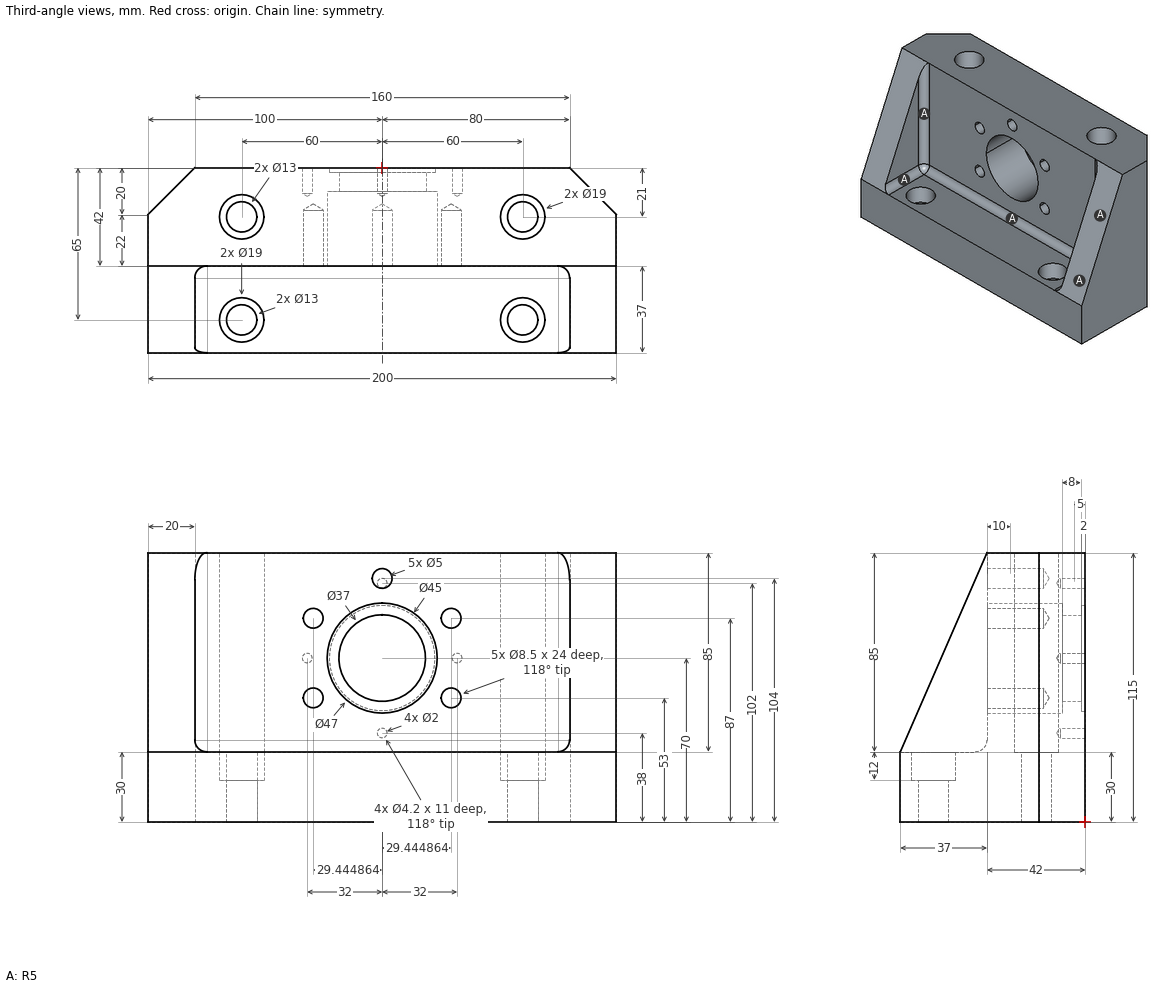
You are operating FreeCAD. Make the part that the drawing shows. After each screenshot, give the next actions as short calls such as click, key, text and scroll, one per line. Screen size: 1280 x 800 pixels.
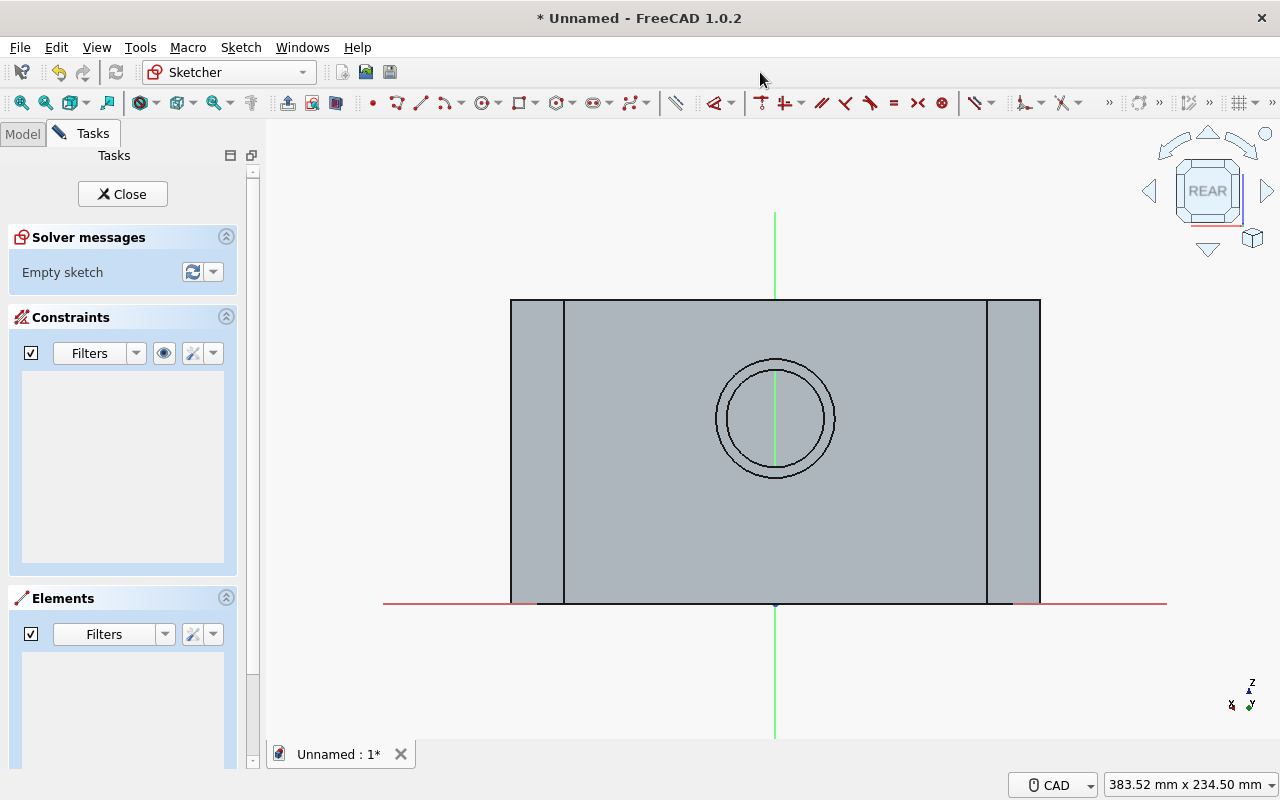
click(336, 104)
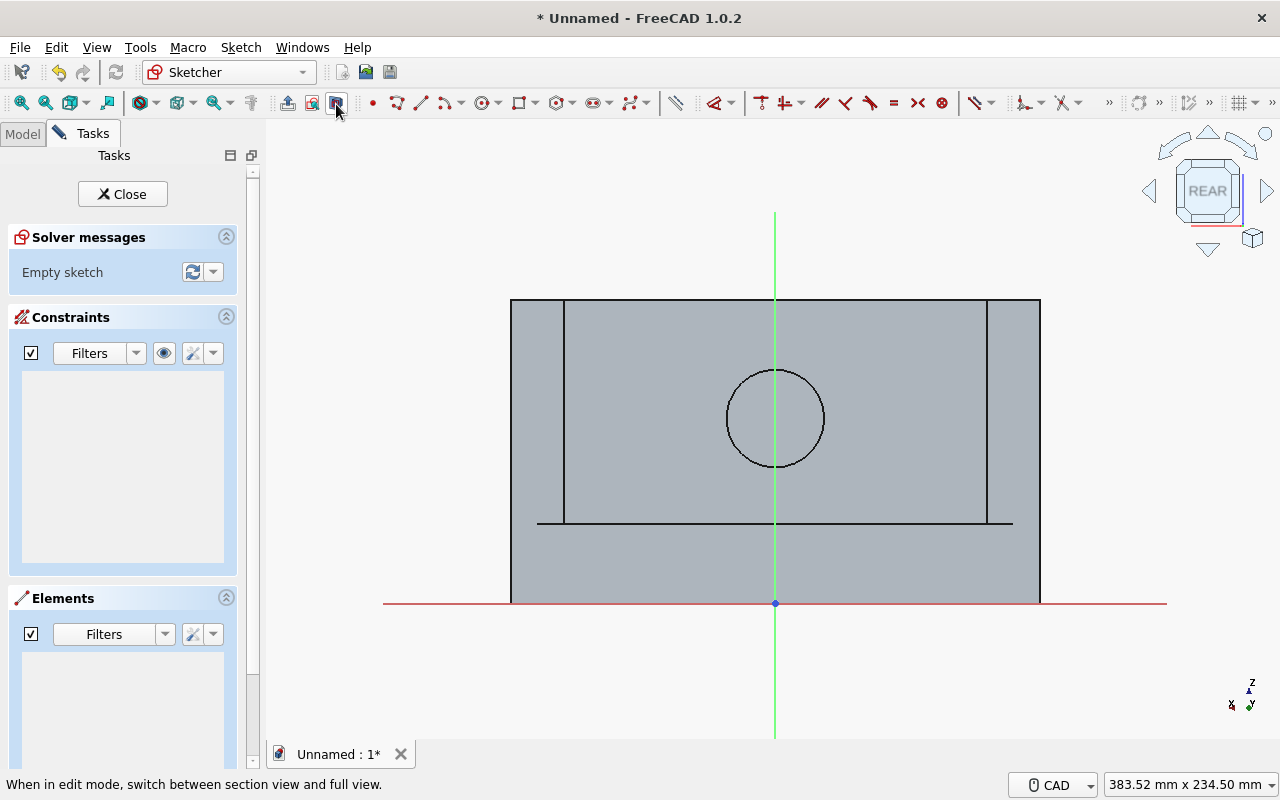
scroll(919, 584, up, 2)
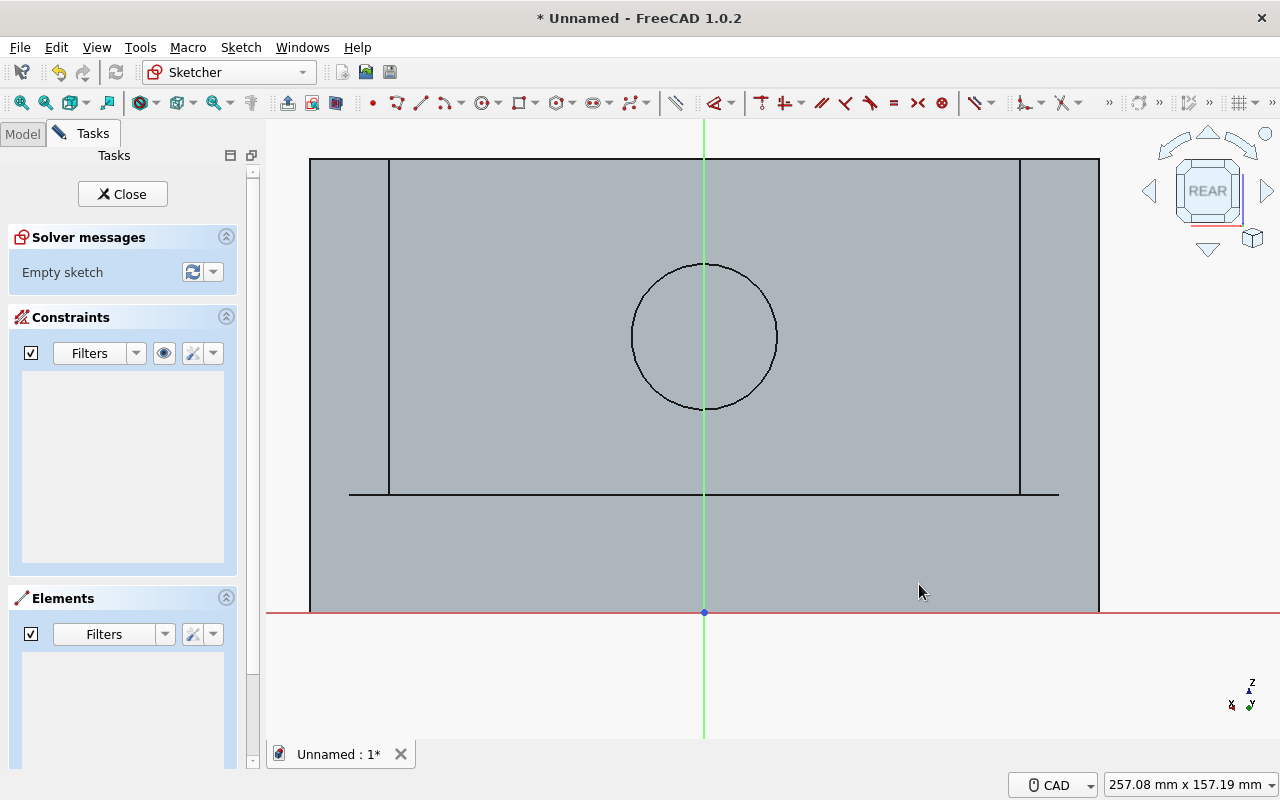
click(482, 104)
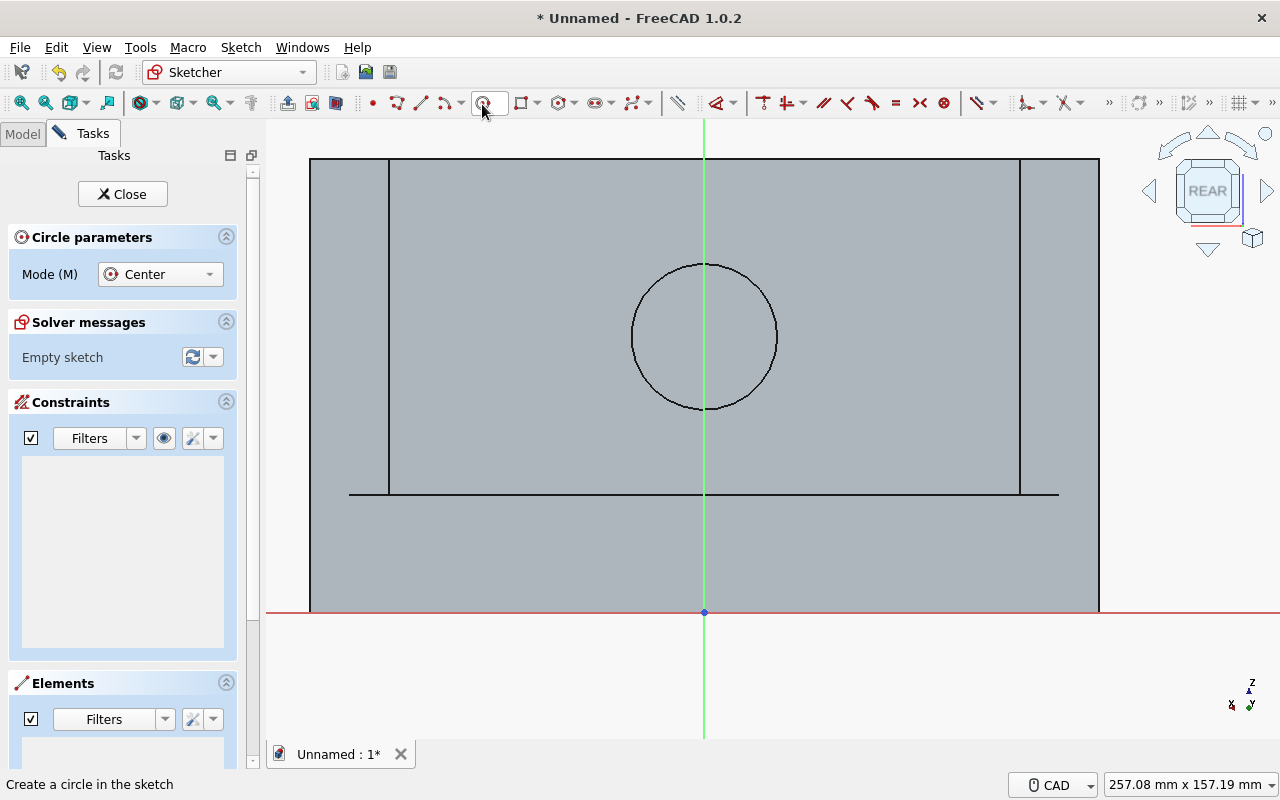
click(704, 337)
move(770, 271)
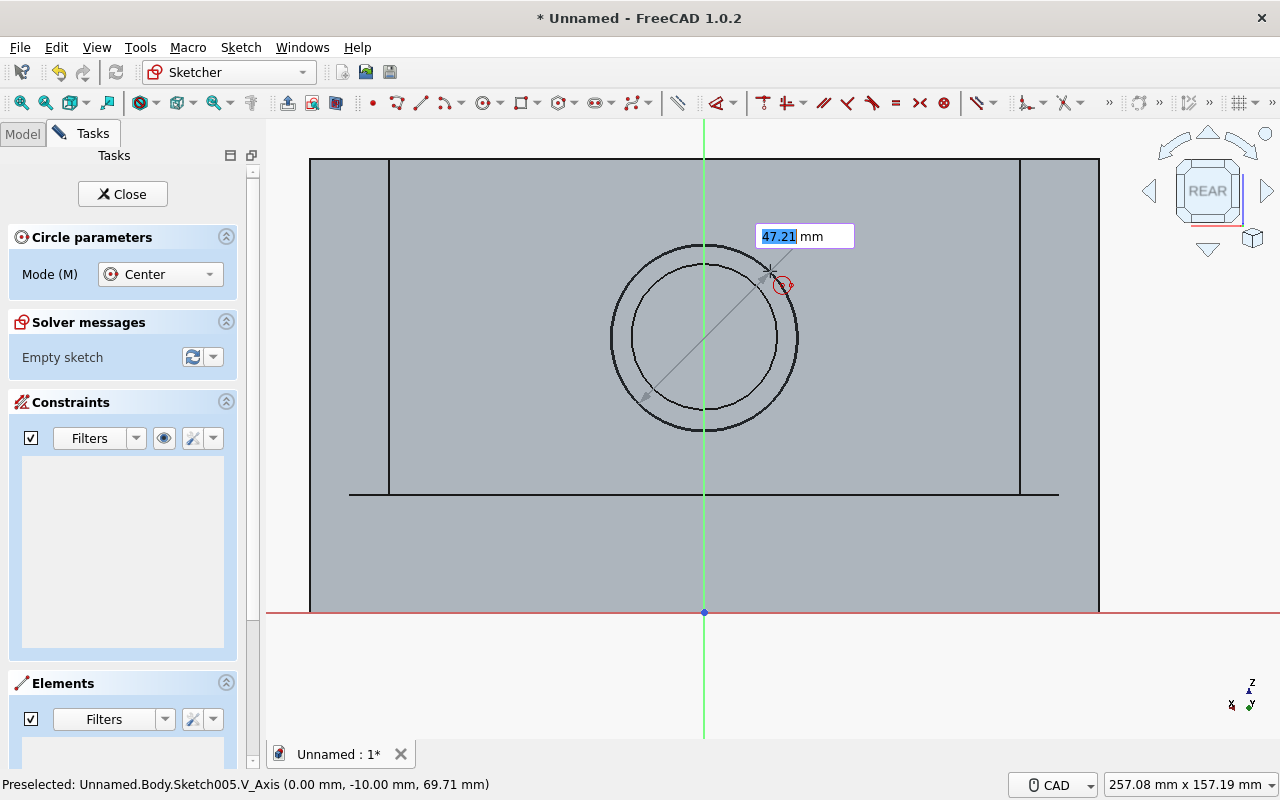
text(47)
key(Return)
key(Escape)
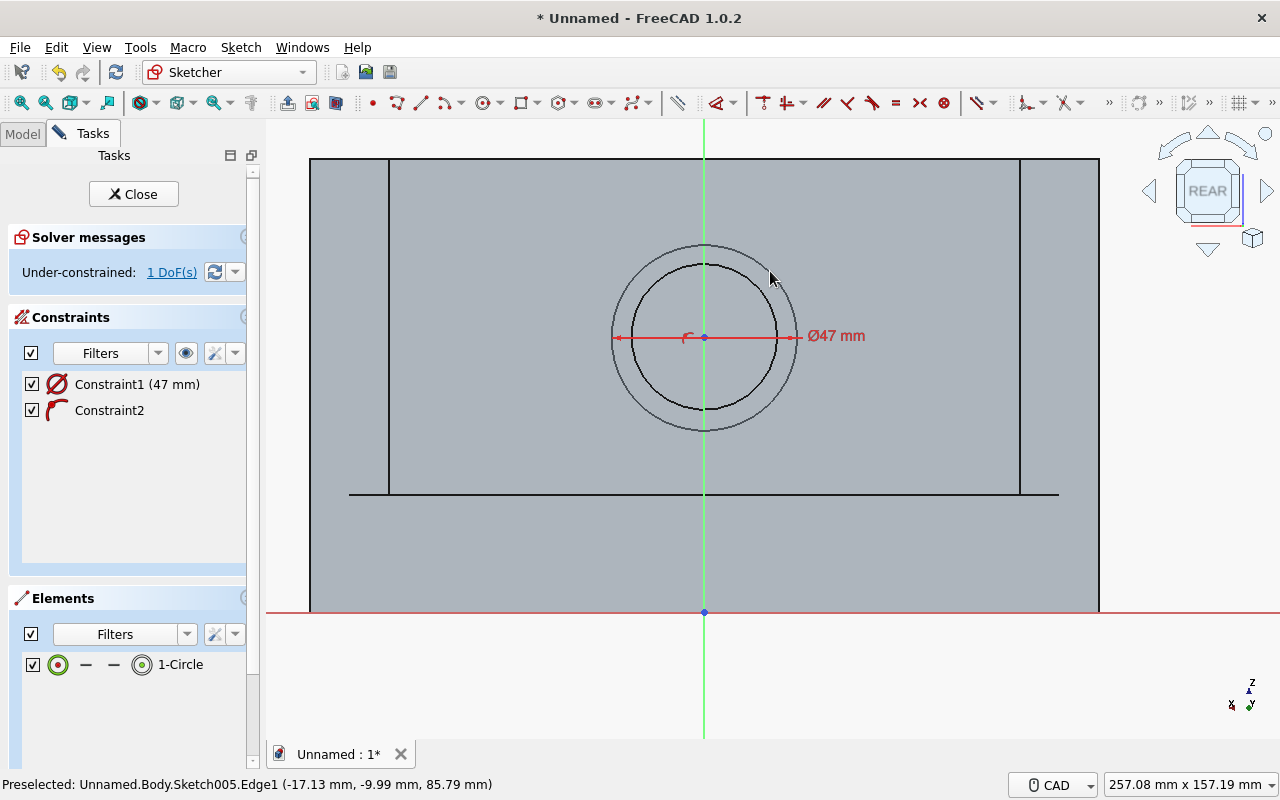
key(d)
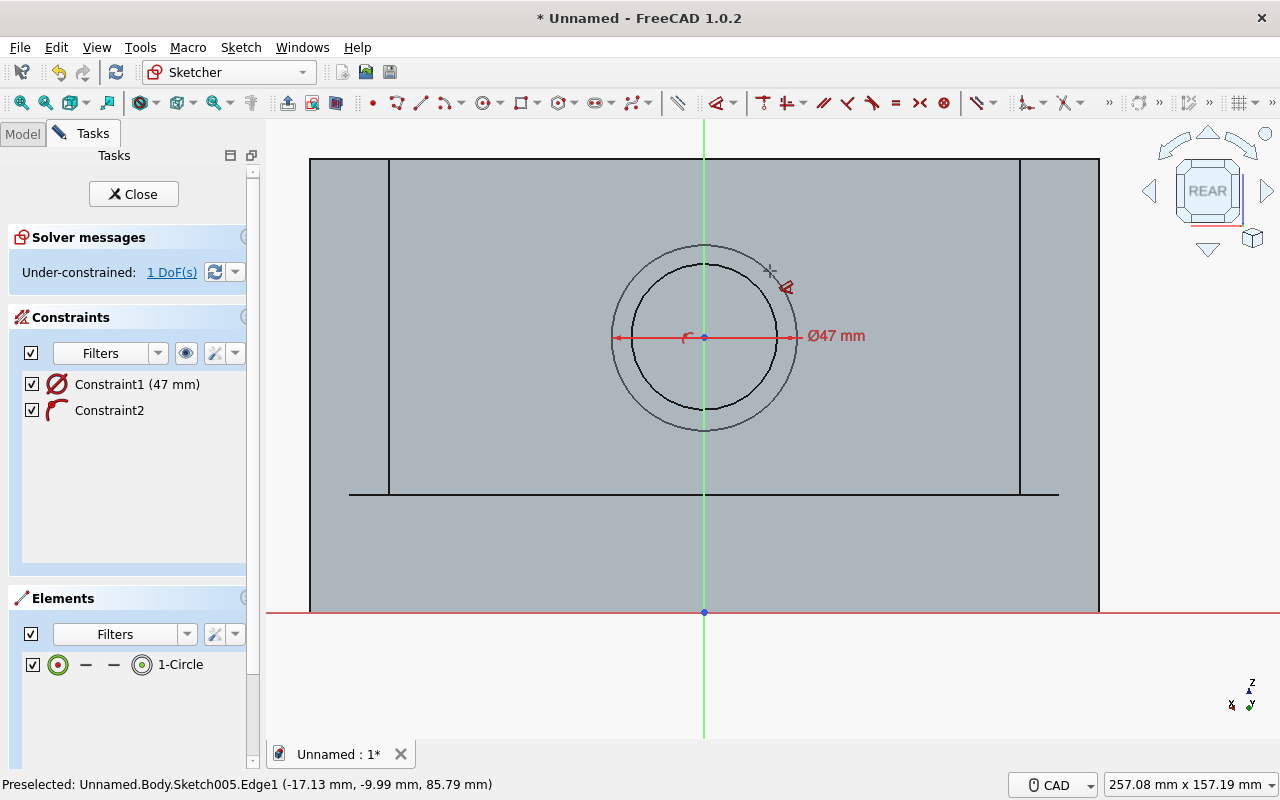
click(704, 338)
click(738, 475)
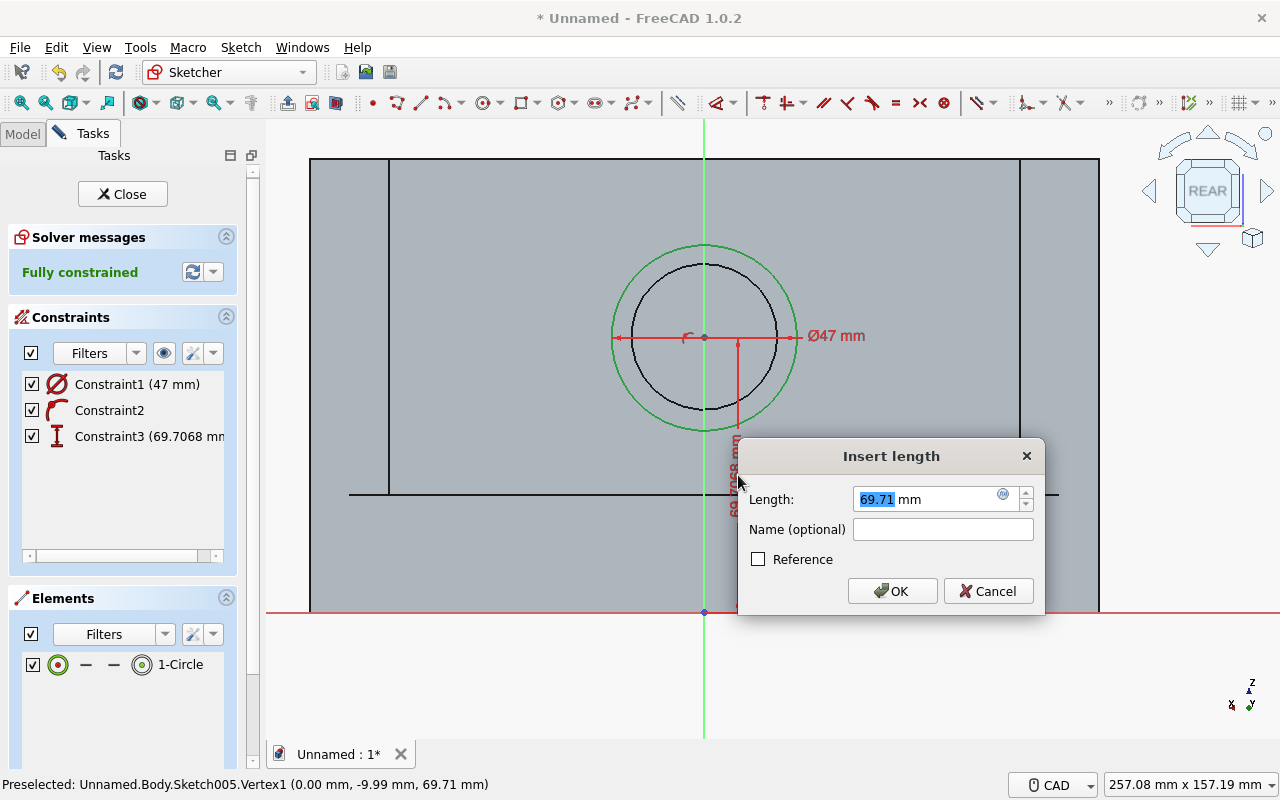
text(70)
key(Return)
key(Escape)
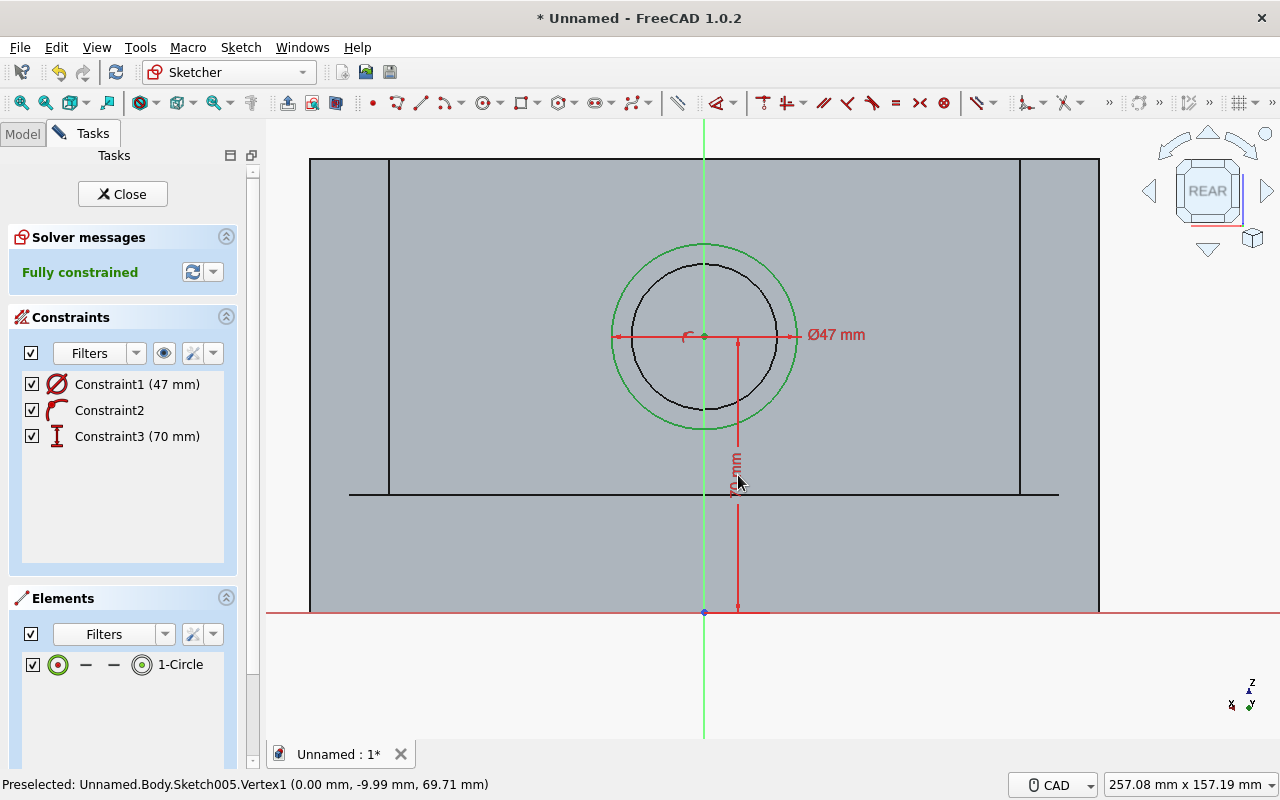
click(123, 194)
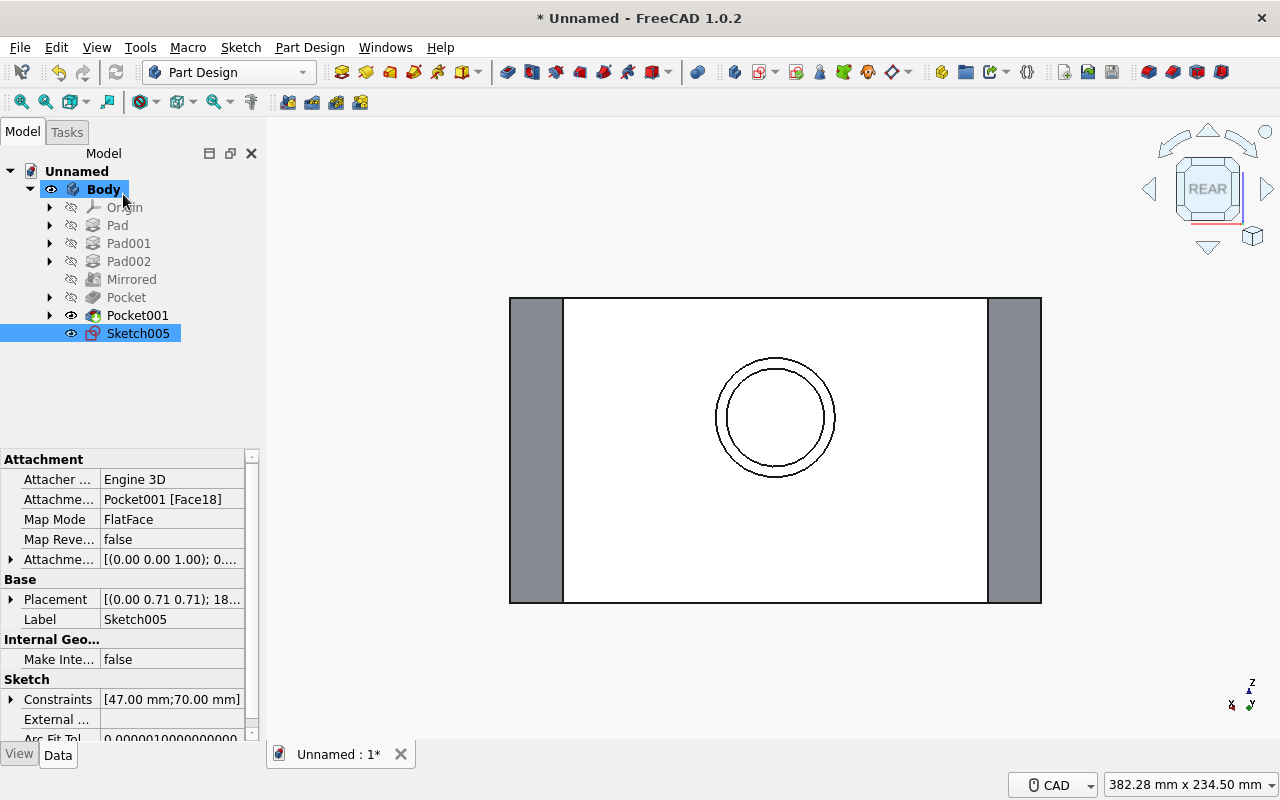
click(508, 72)